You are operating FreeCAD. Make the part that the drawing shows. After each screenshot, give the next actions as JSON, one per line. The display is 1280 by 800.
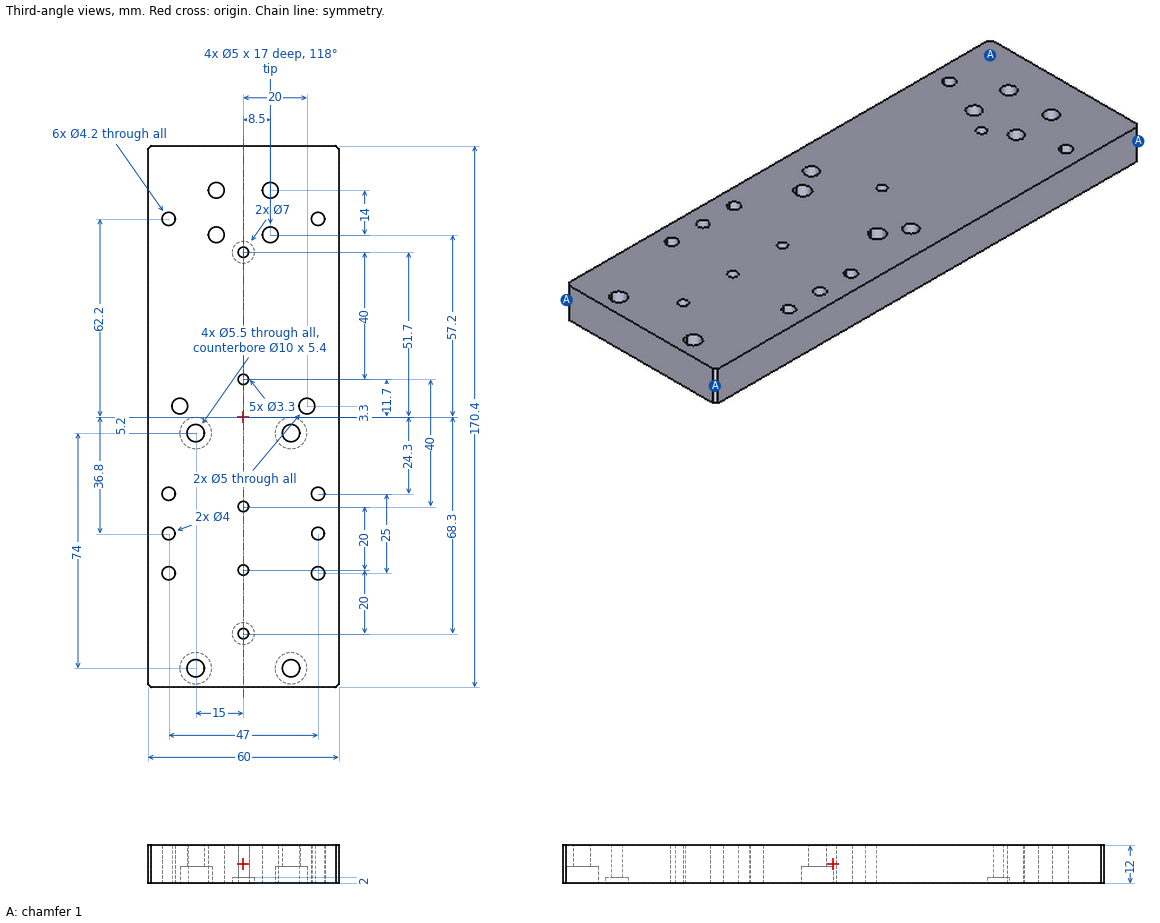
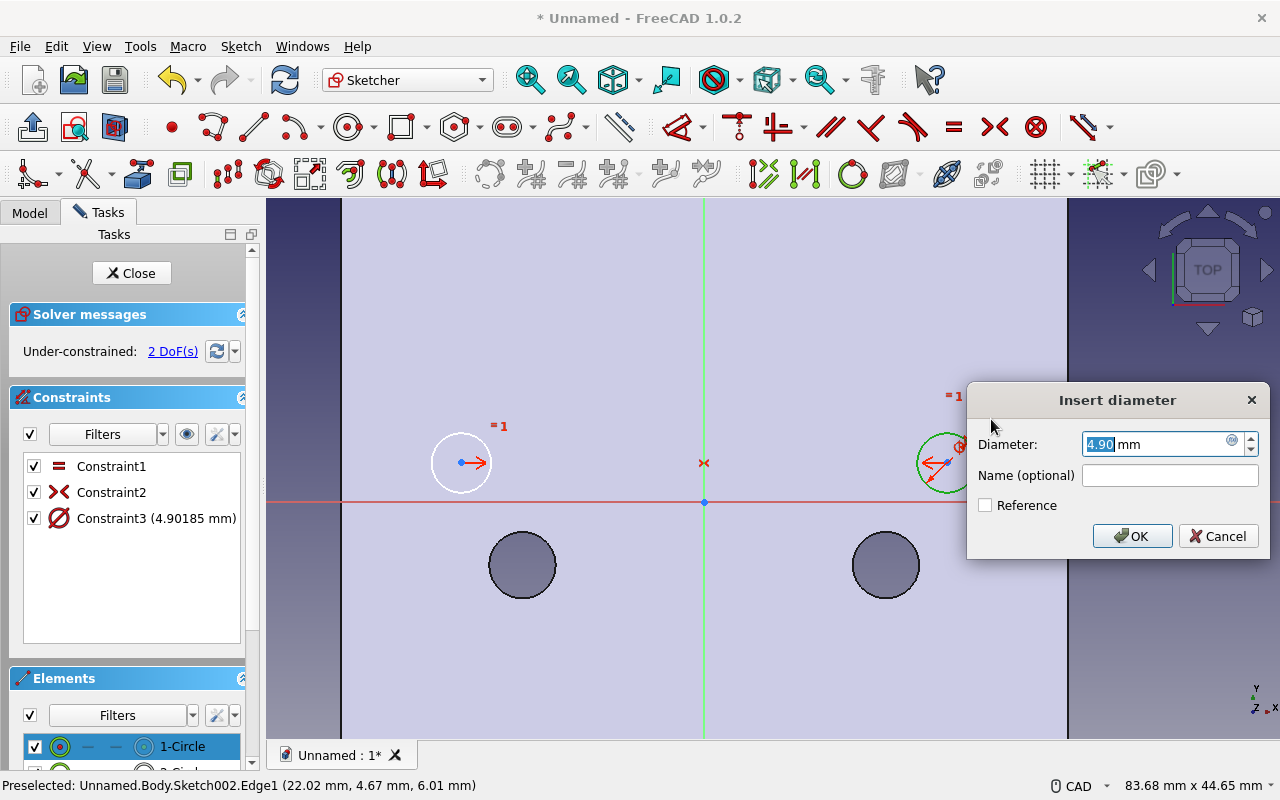
{"action": "type", "text": "5"}
{"action": "key", "text": "Return"}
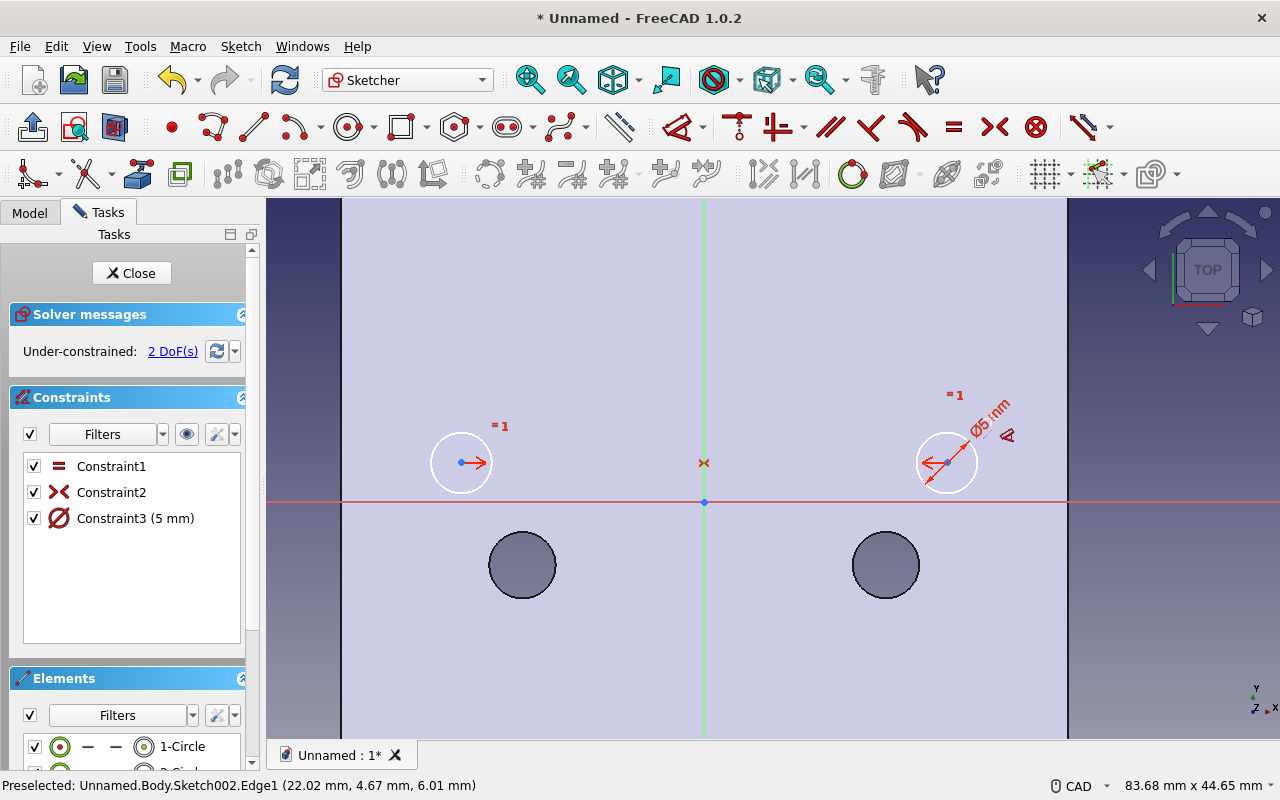
{"action": "left_click", "coordinate": [947, 463]}
{"action": "left_click", "coordinate": [826, 536]}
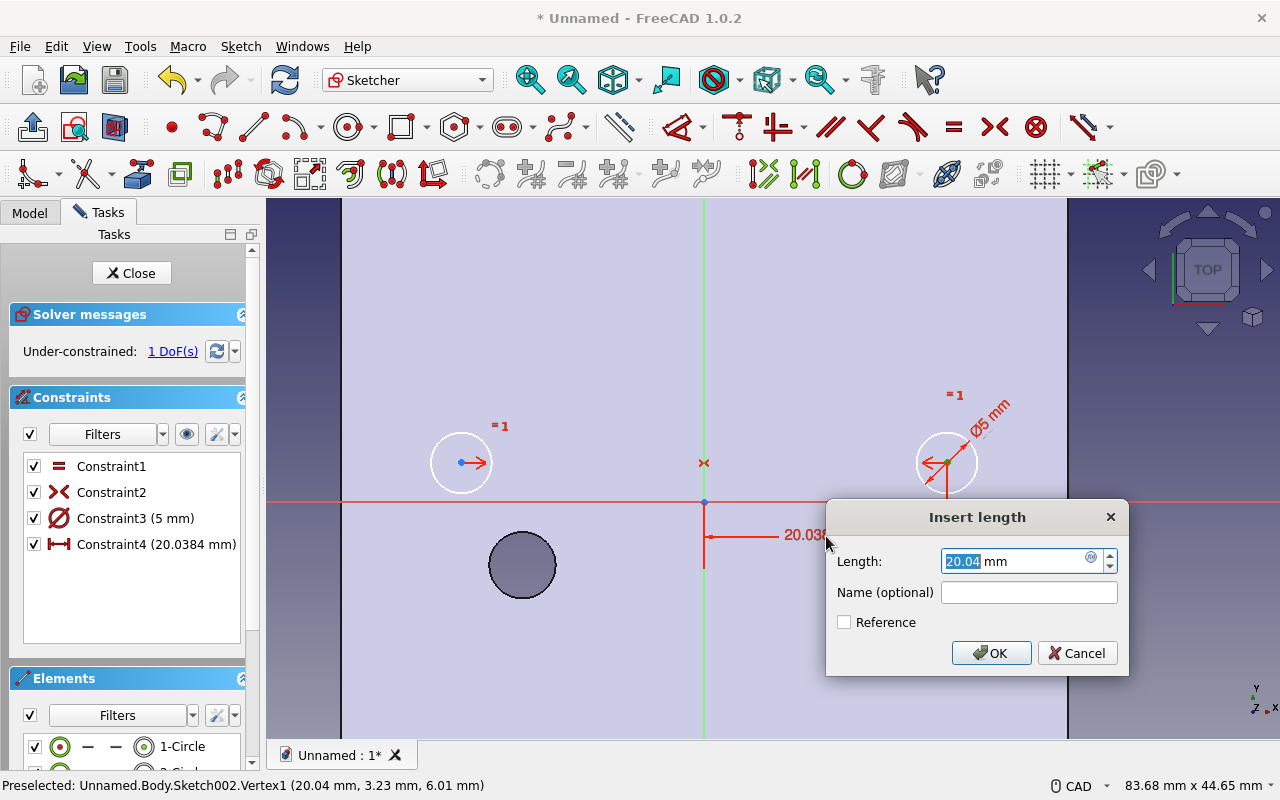
{"action": "type", "text": "20"}
{"action": "key", "text": "Return"}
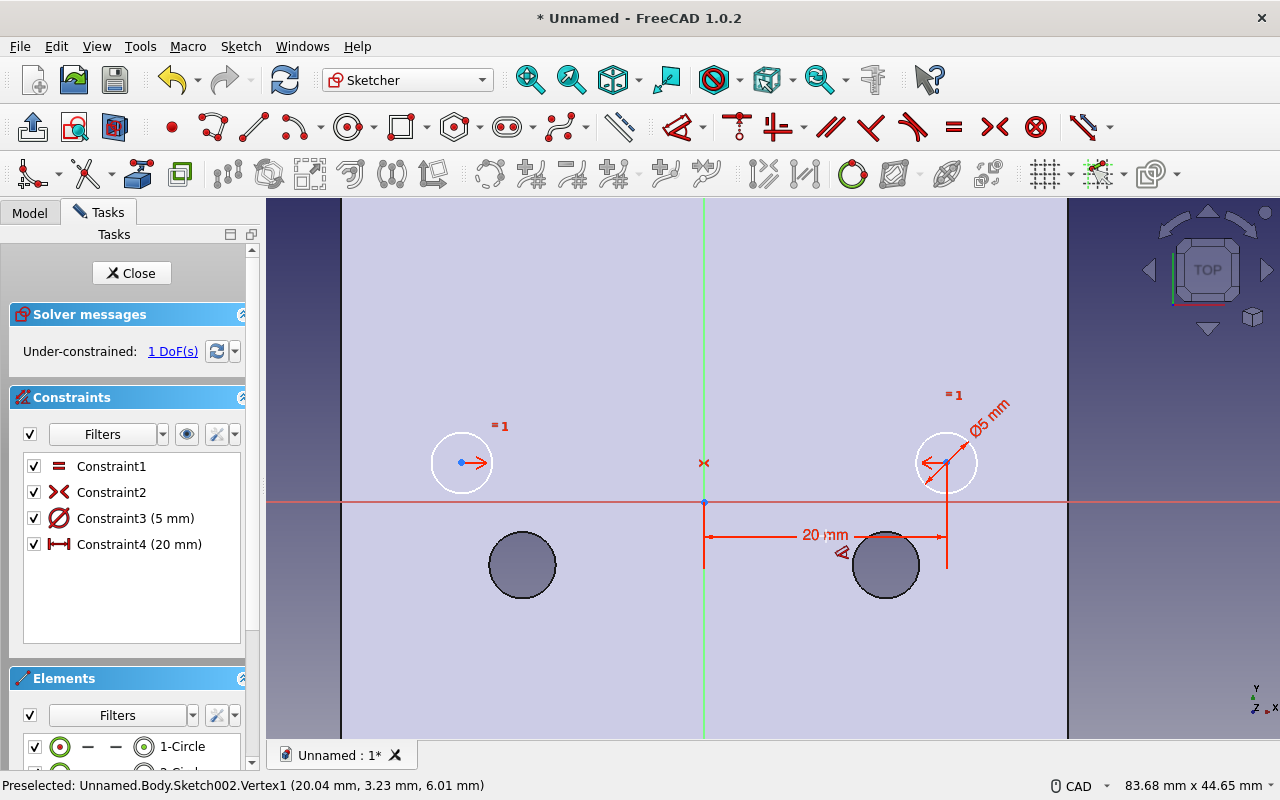
{"action": "left_click", "coordinate": [947, 463]}
{"action": "left_click", "coordinate": [670, 483]}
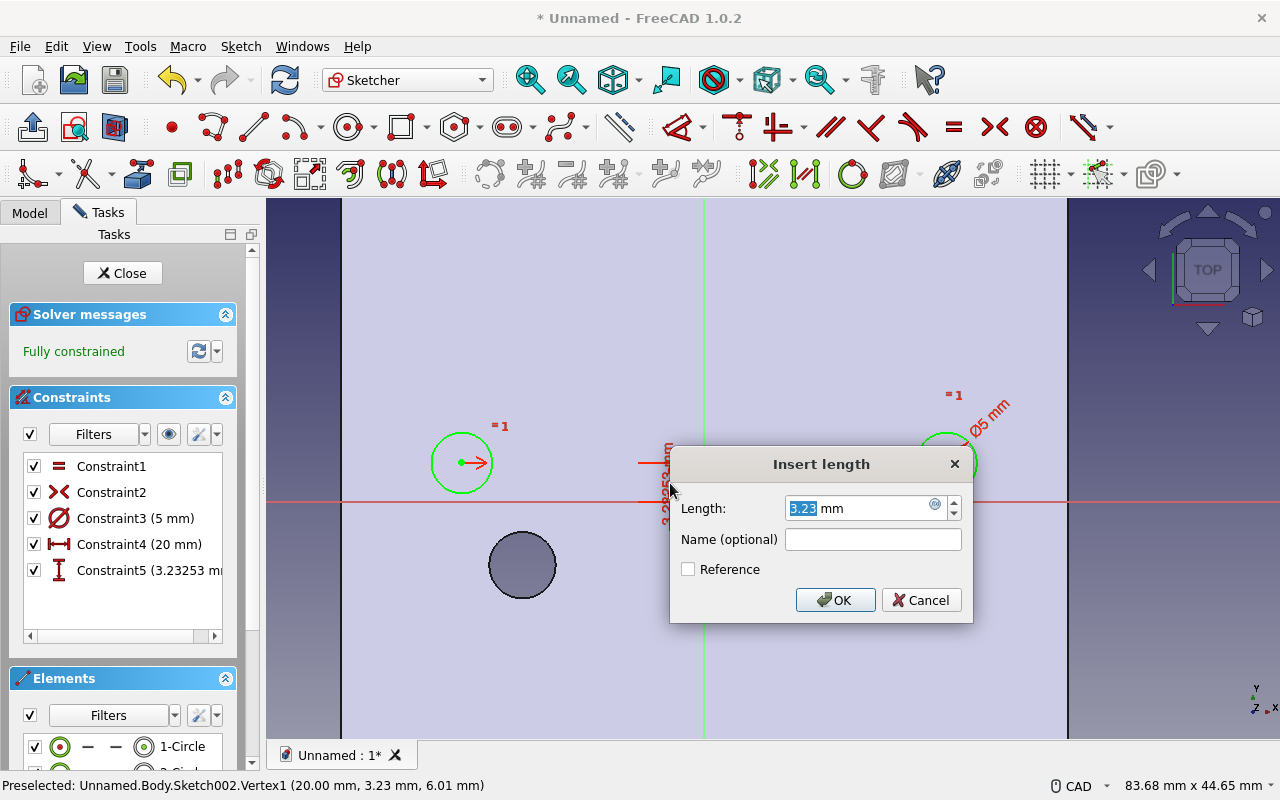
{"action": "type", "text": "3.3"}
{"action": "key", "text": "Return"}
{"action": "key", "text": "Escape"}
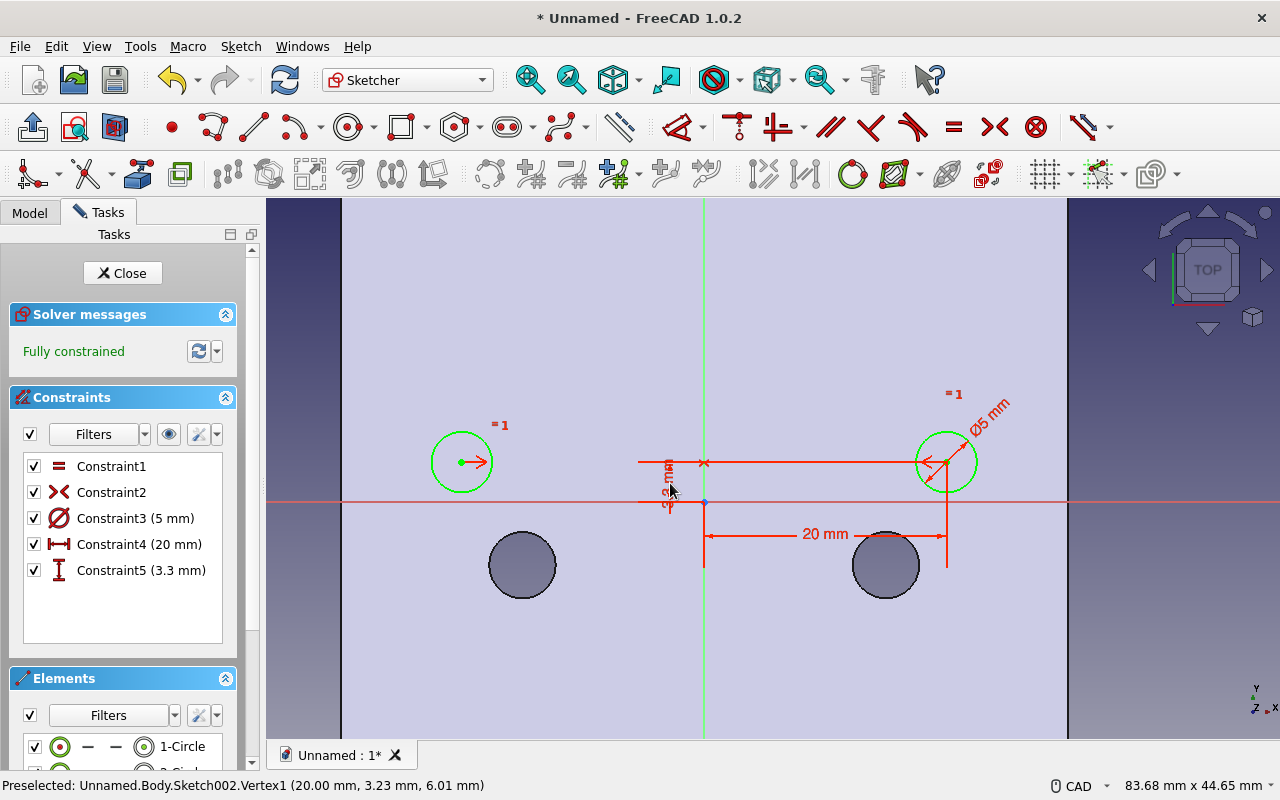
{"action": "left_click", "coordinate": [123, 273]}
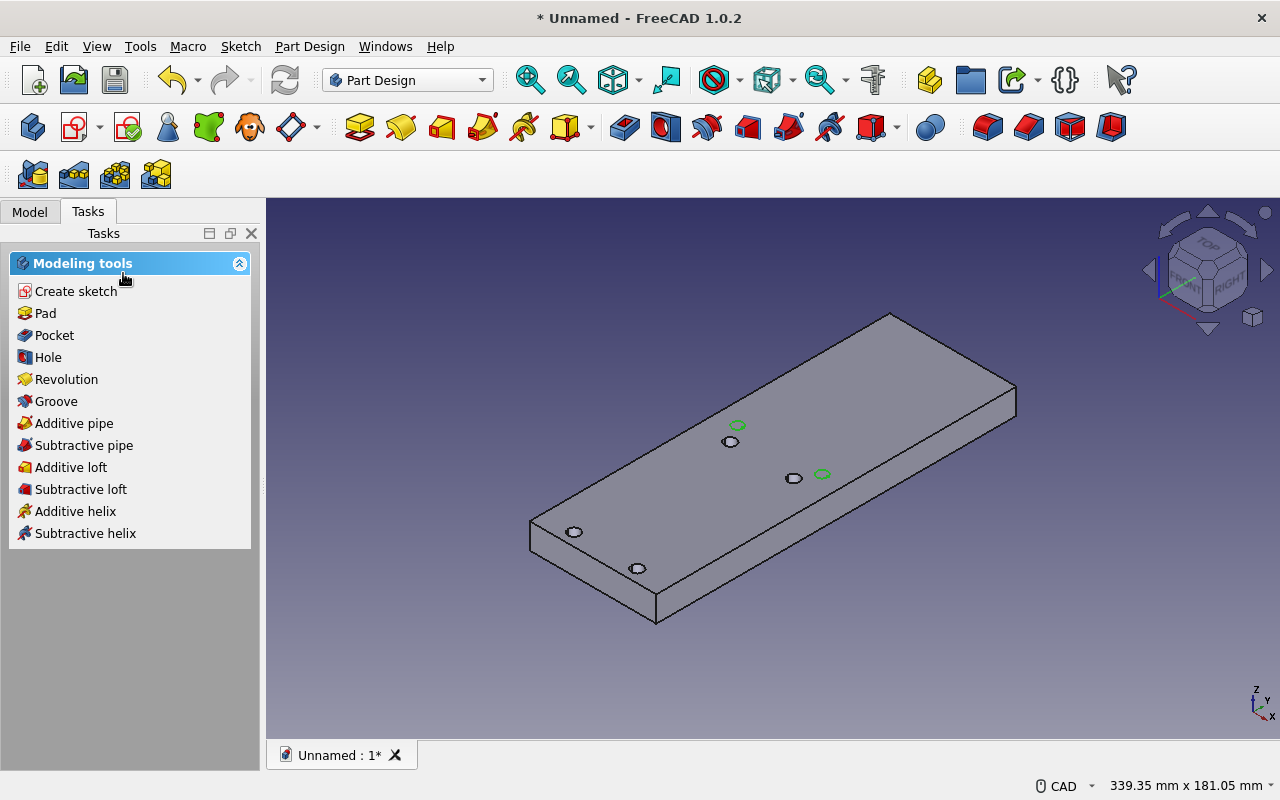
{"action": "left_click", "coordinate": [666, 128]}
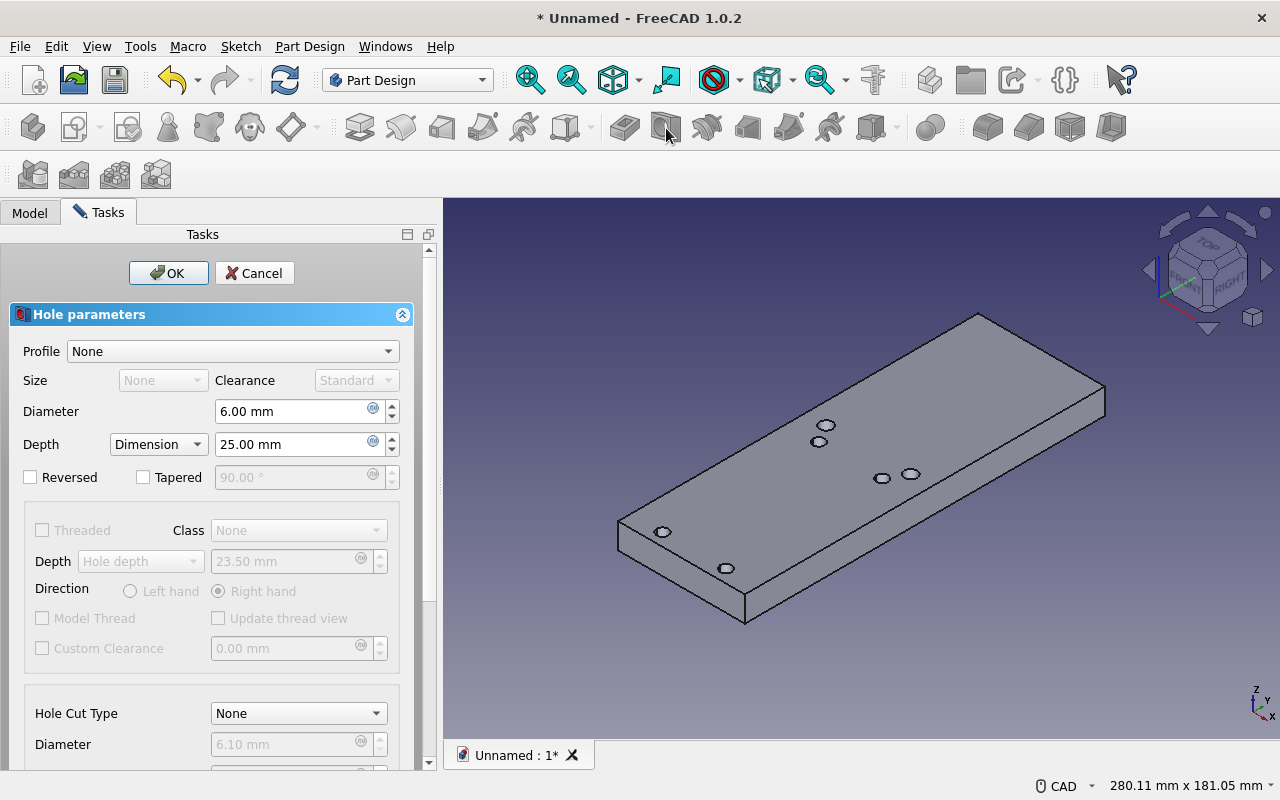
{"action": "triple_click", "coordinate": [300, 412]}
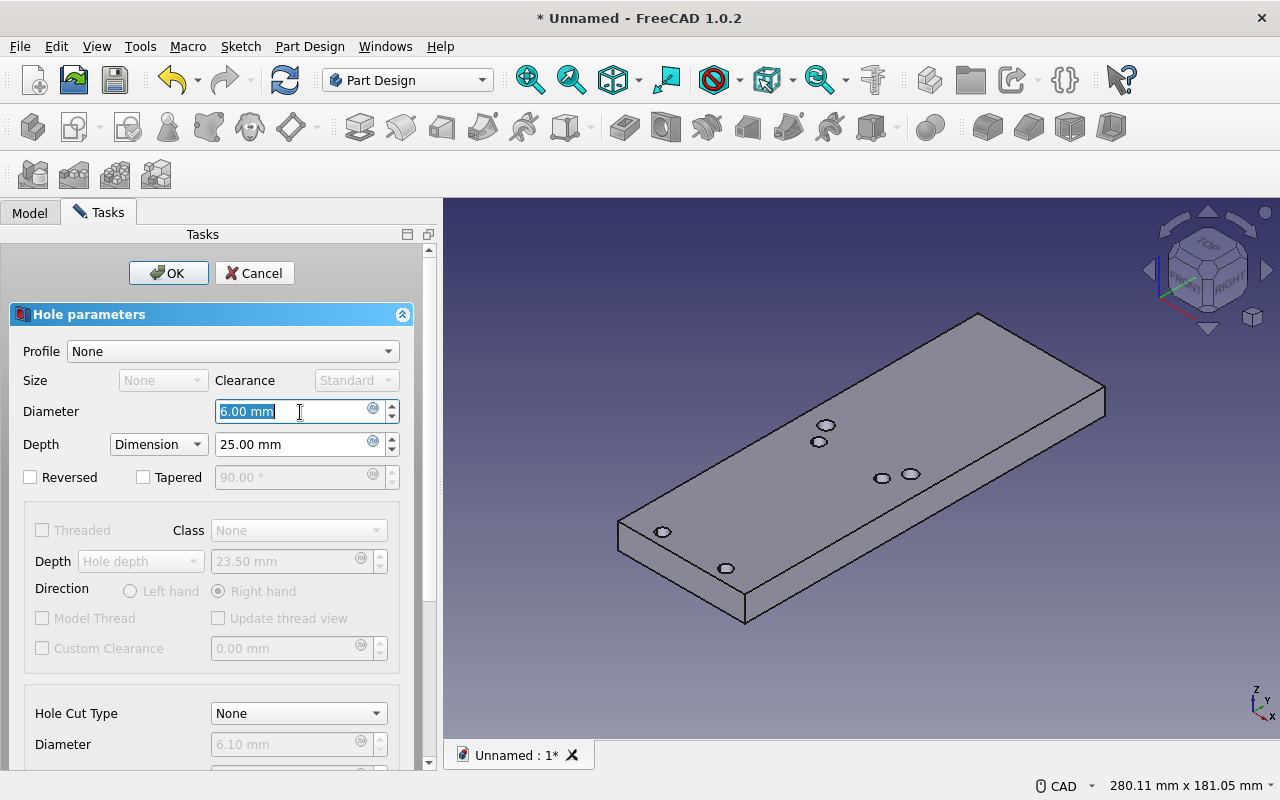
{"action": "type", "text": "5"}
{"action": "key", "text": "Tab"}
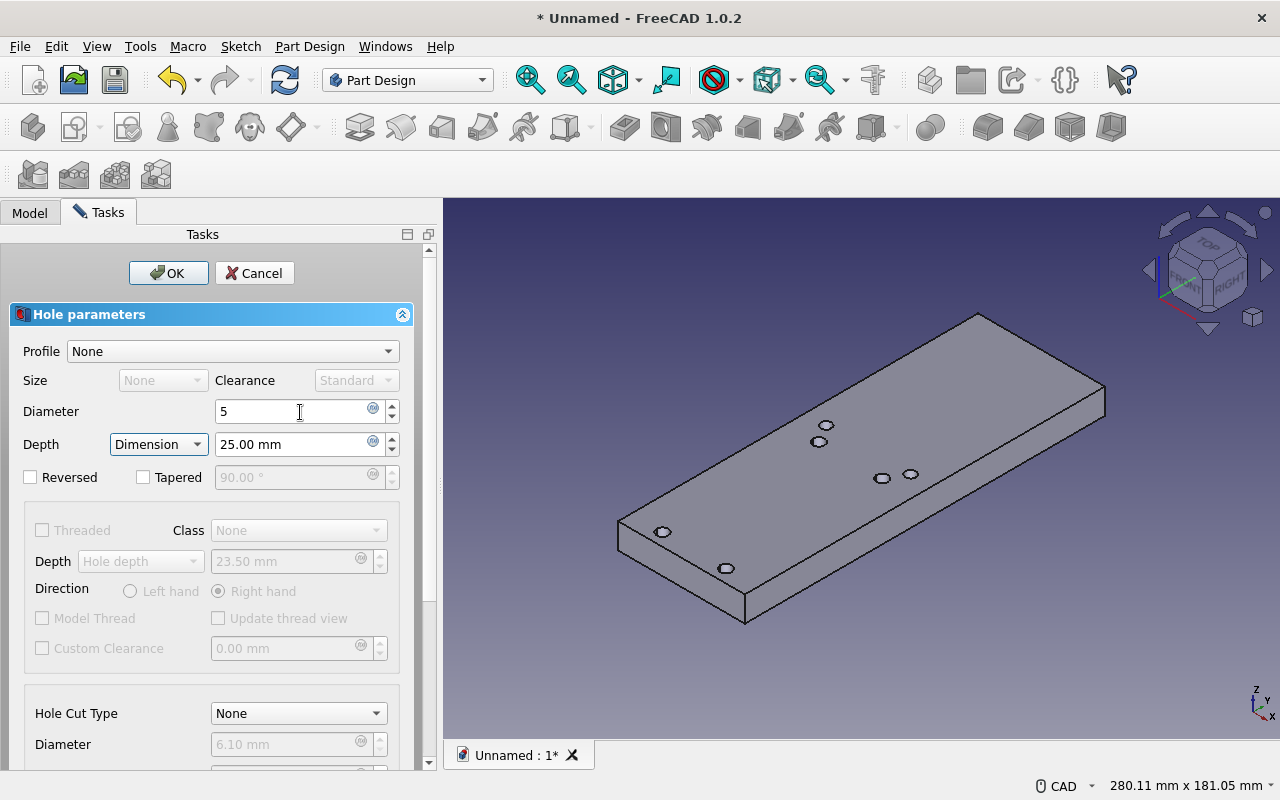
{"action": "left_click", "coordinate": [160, 444]}